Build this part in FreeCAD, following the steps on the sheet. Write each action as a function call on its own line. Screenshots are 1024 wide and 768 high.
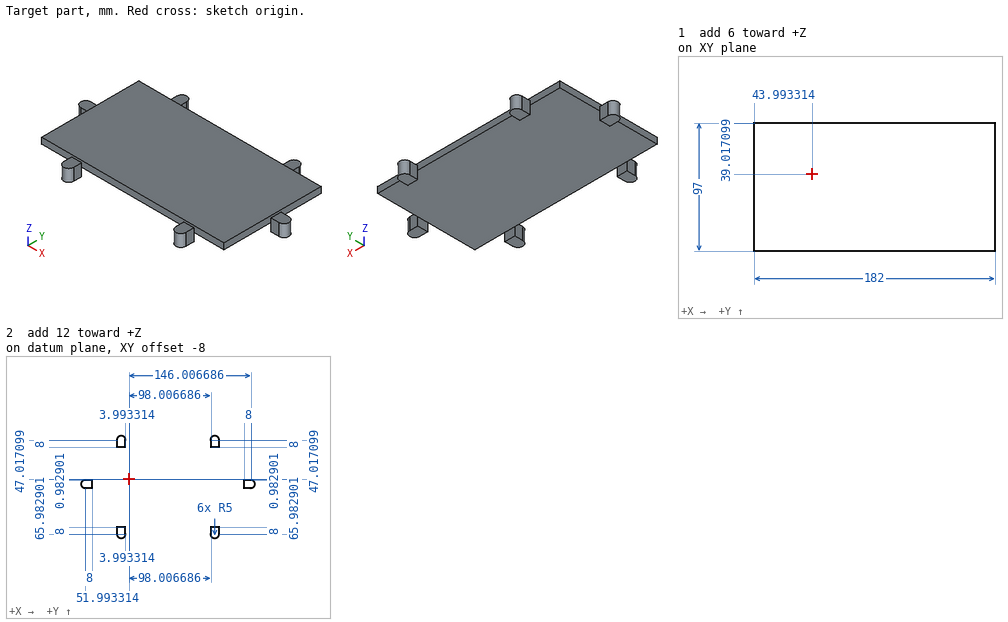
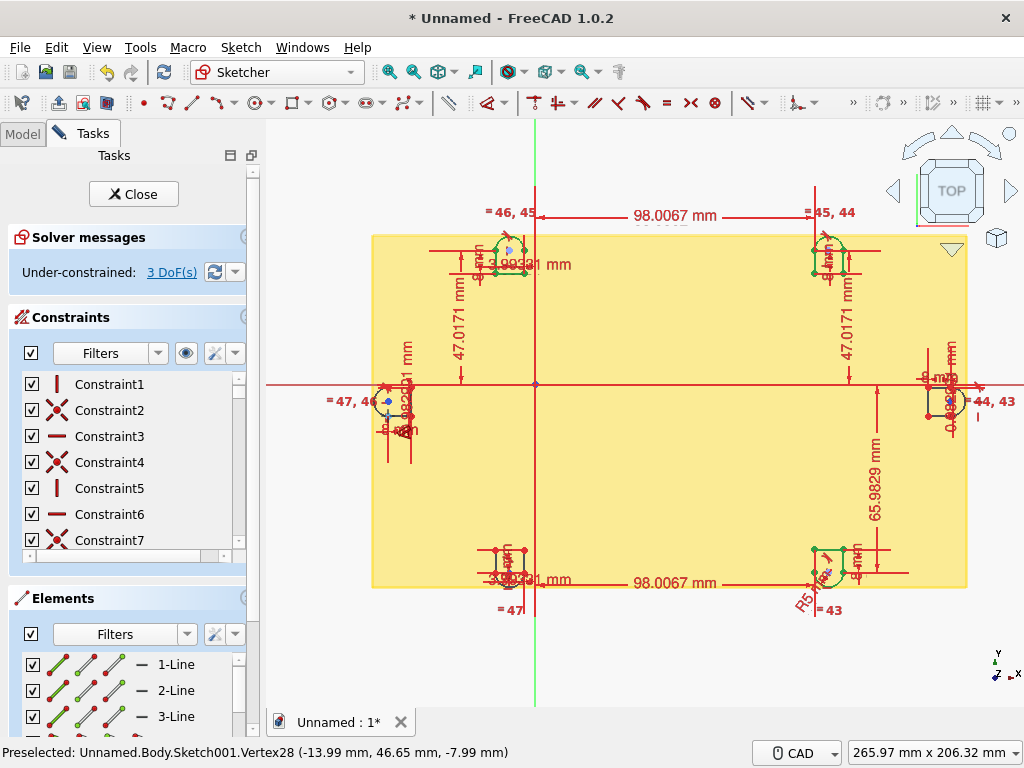
click(388, 416)
click(462, 351)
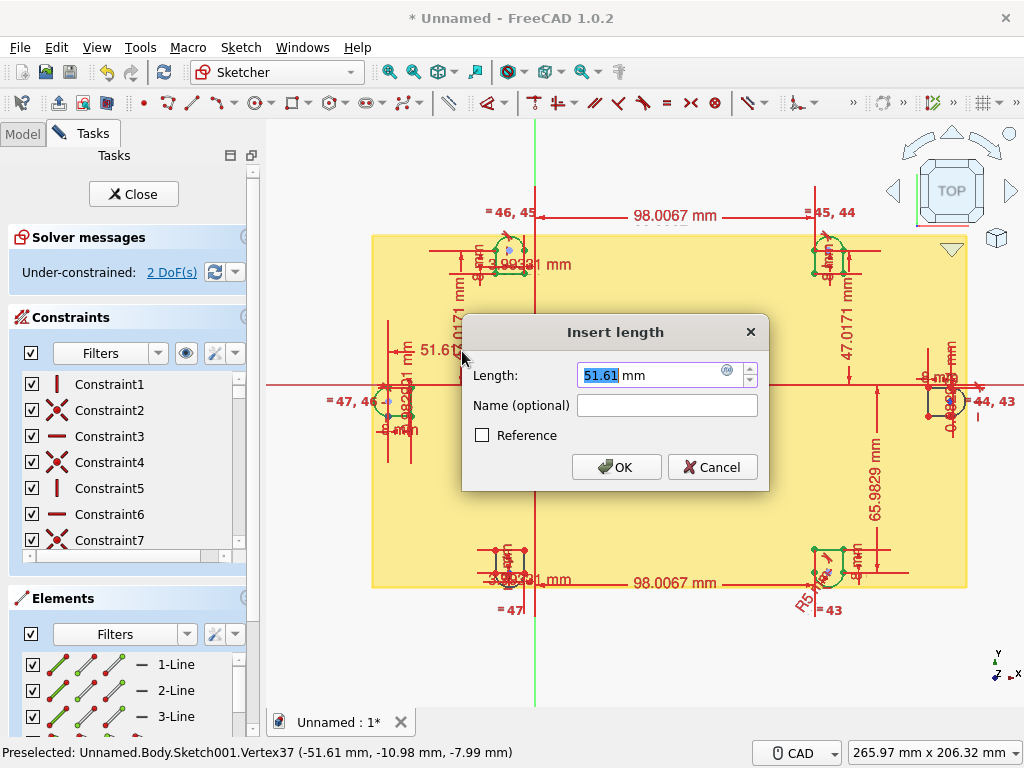
text(51.993314)
key(Return)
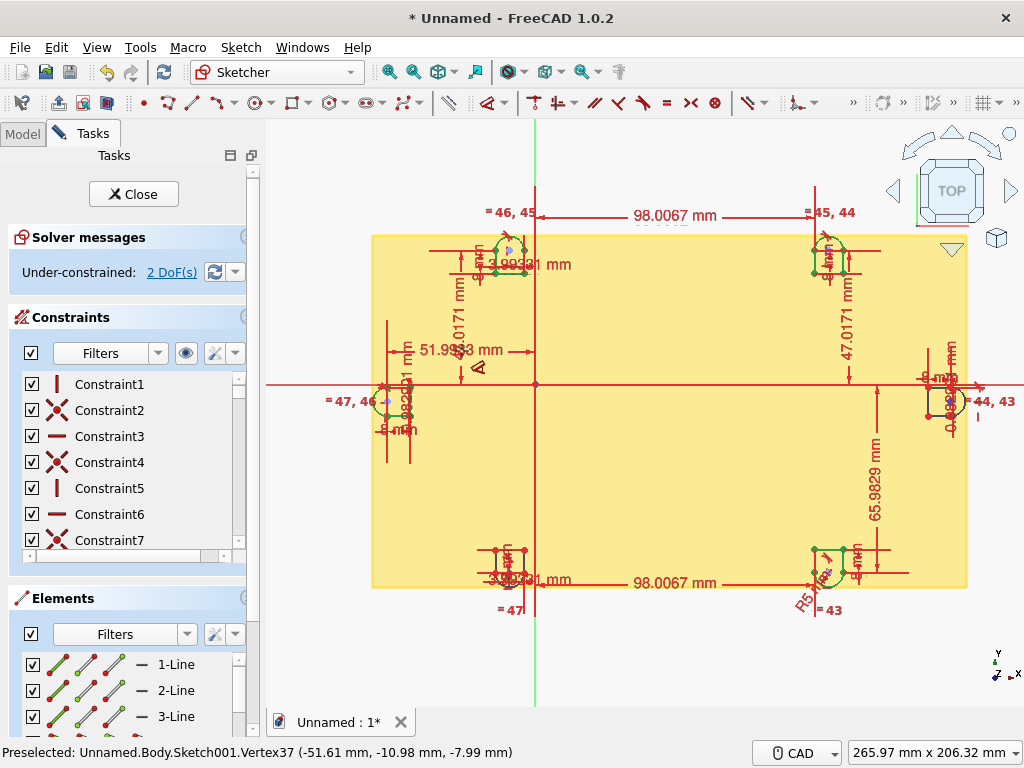
click(524, 573)
click(490, 479)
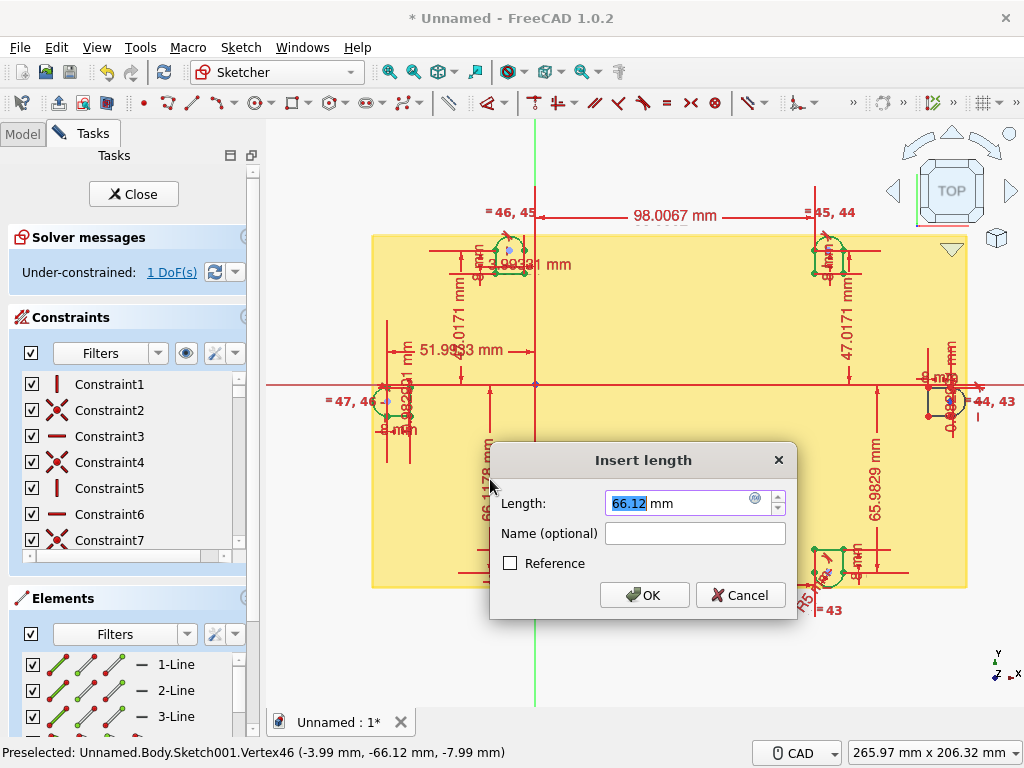
text(65.982901)
key(Return)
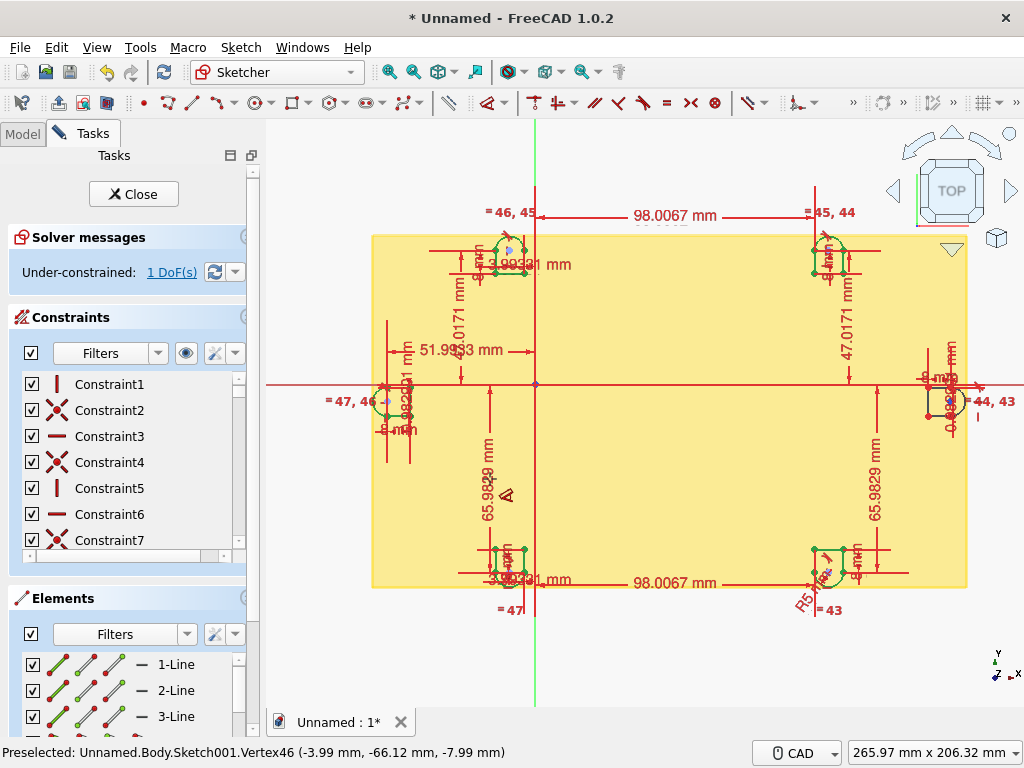
scroll(388, 416, down, 2)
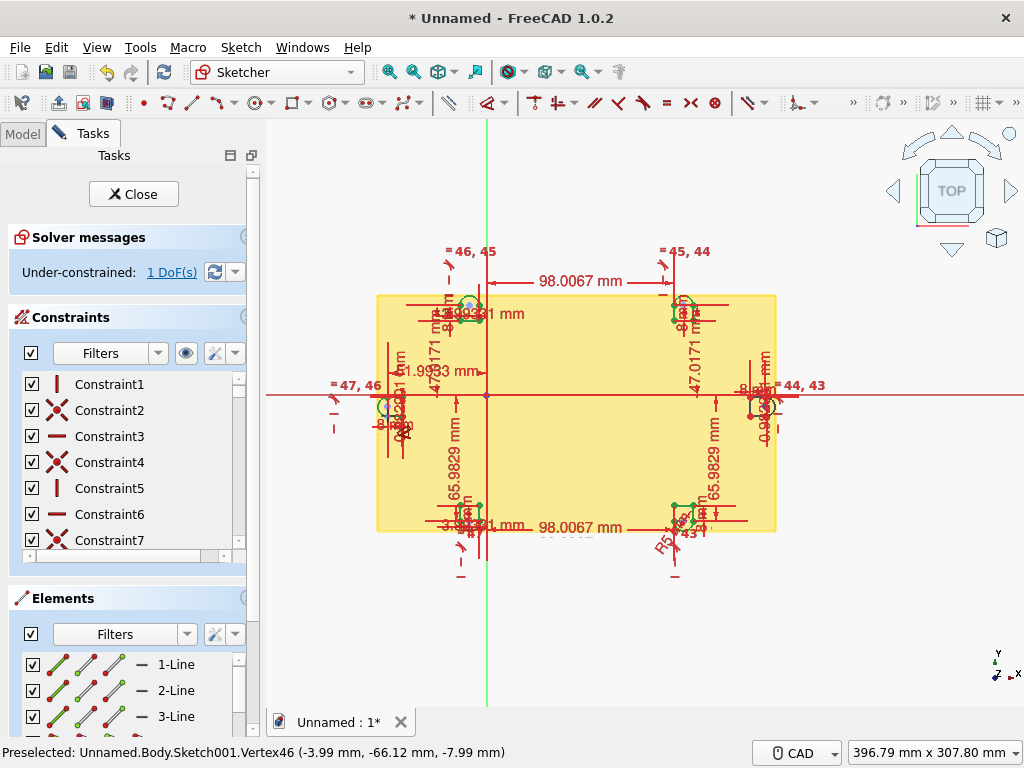
scroll(765, 397, up, 2)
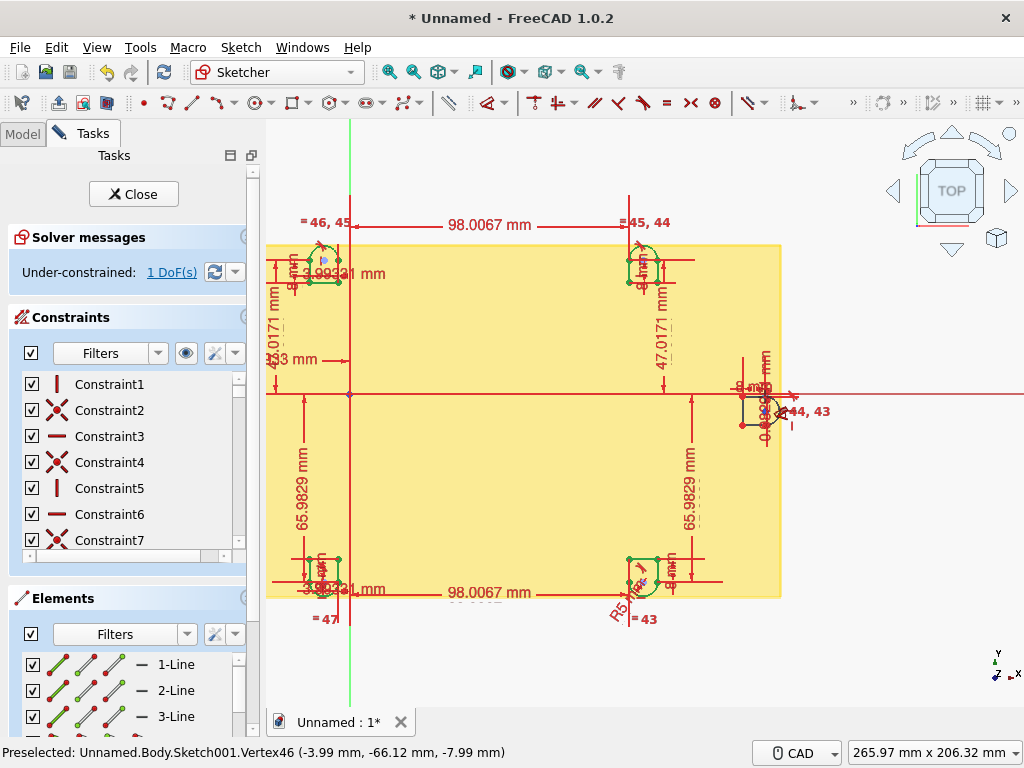
click(765, 397)
click(558, 360)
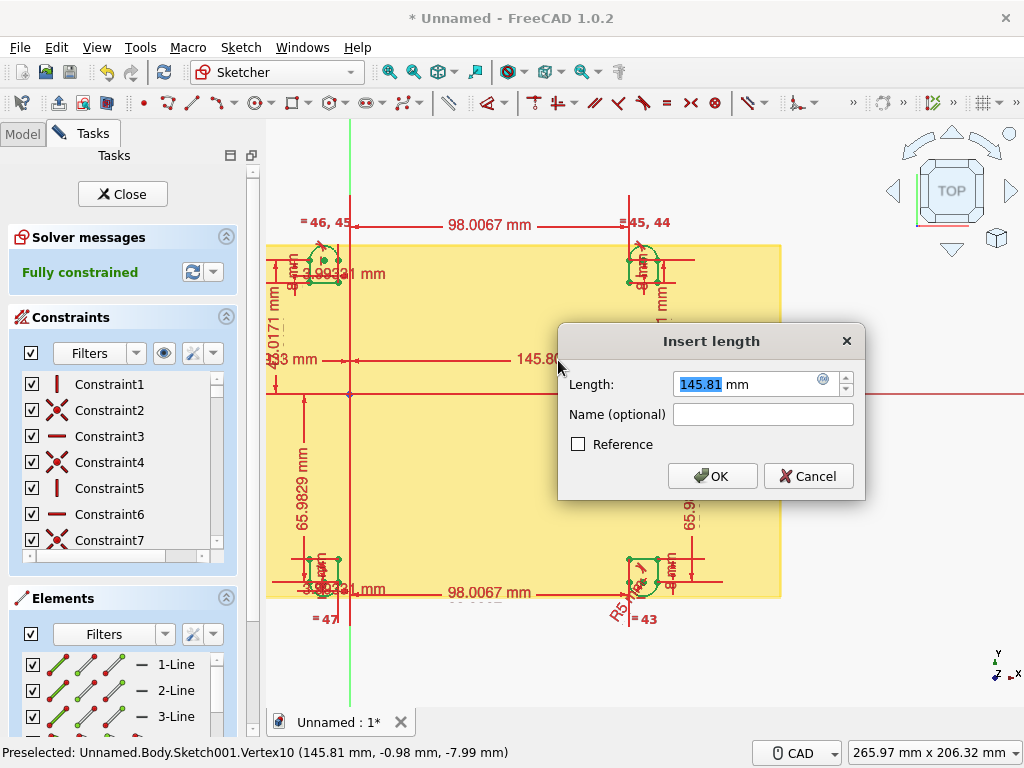
text(146.006686)
key(Return)
key(Escape)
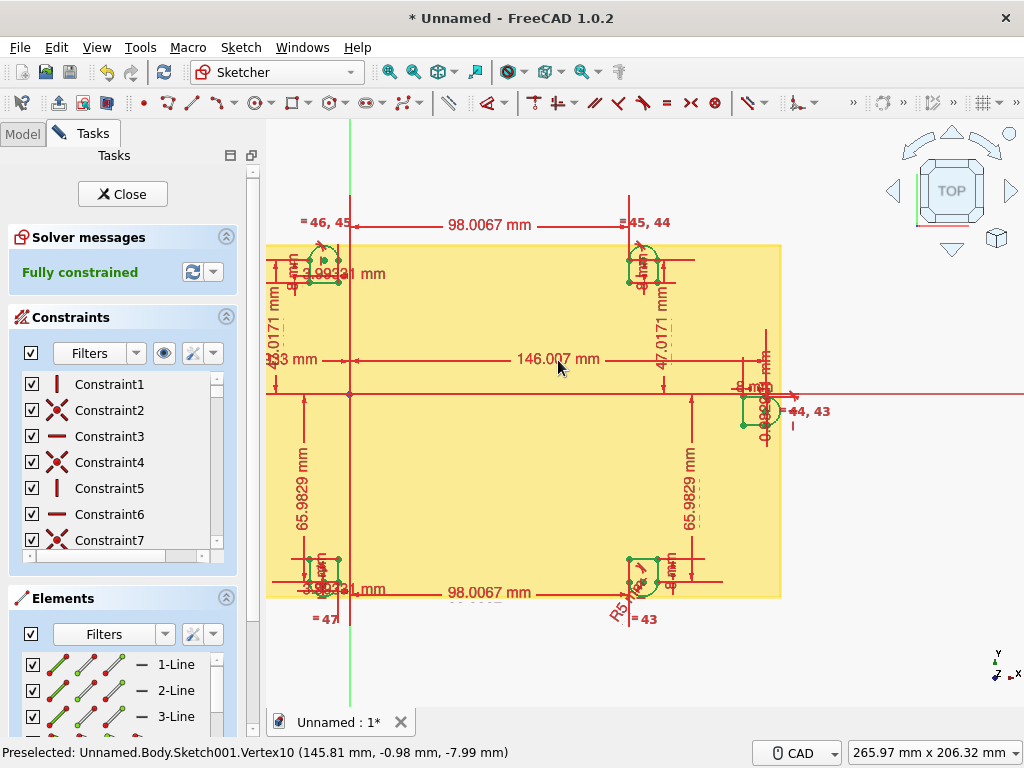
click(123, 194)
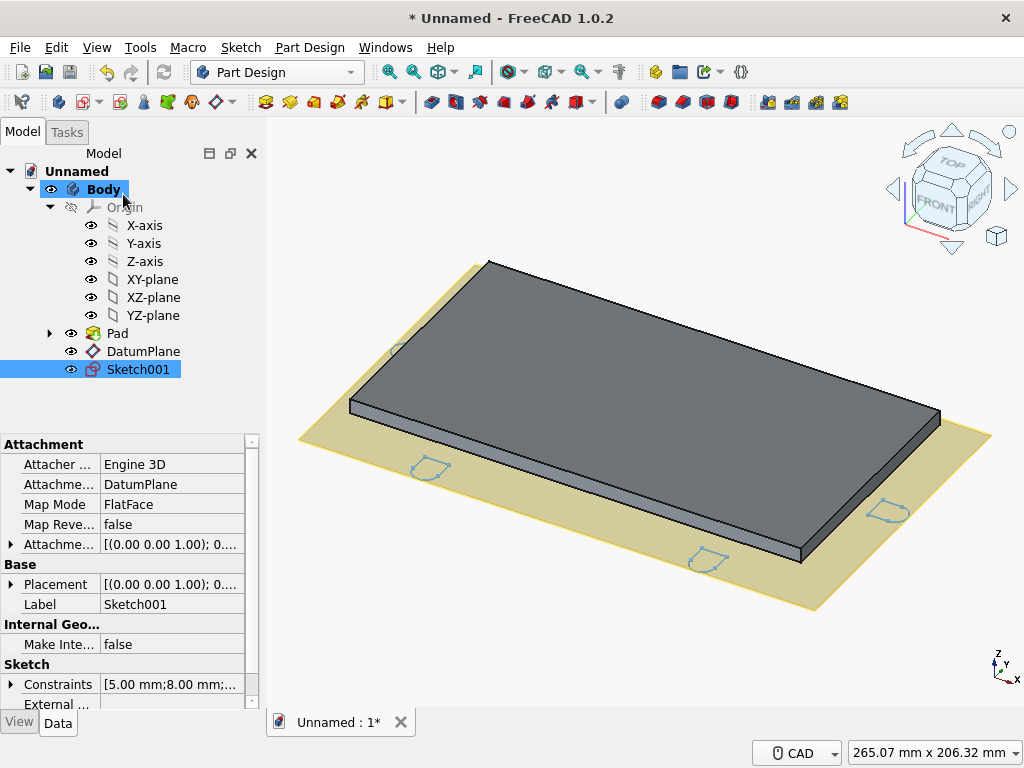
click(266, 102)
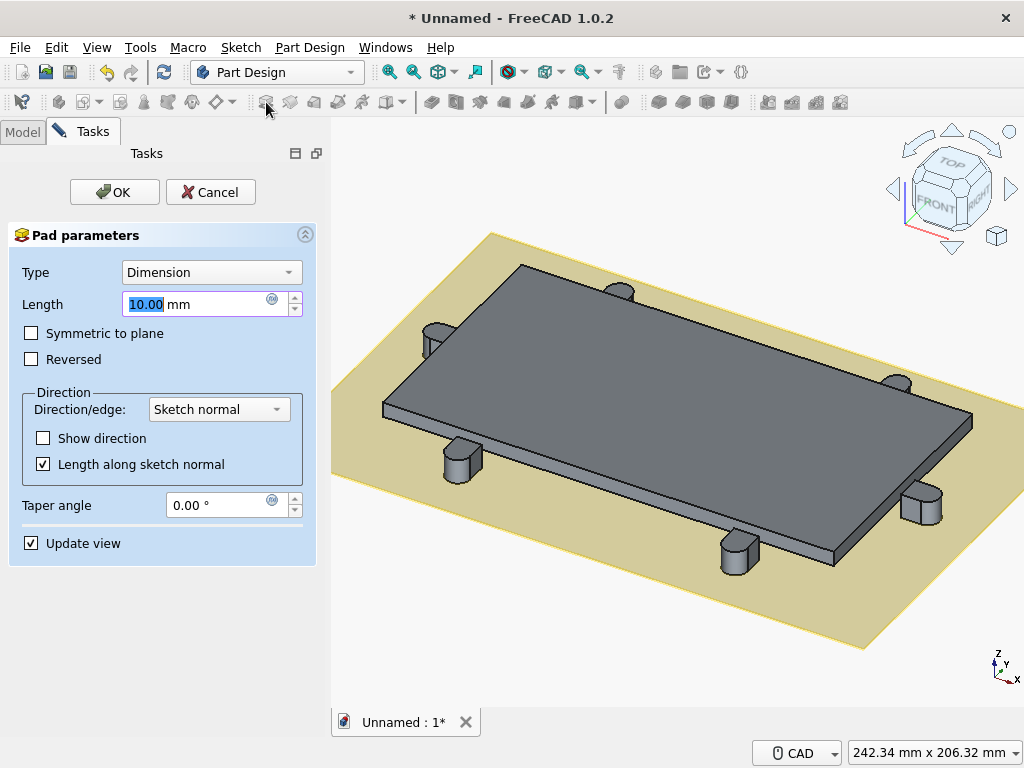
text(12)
key(Tab)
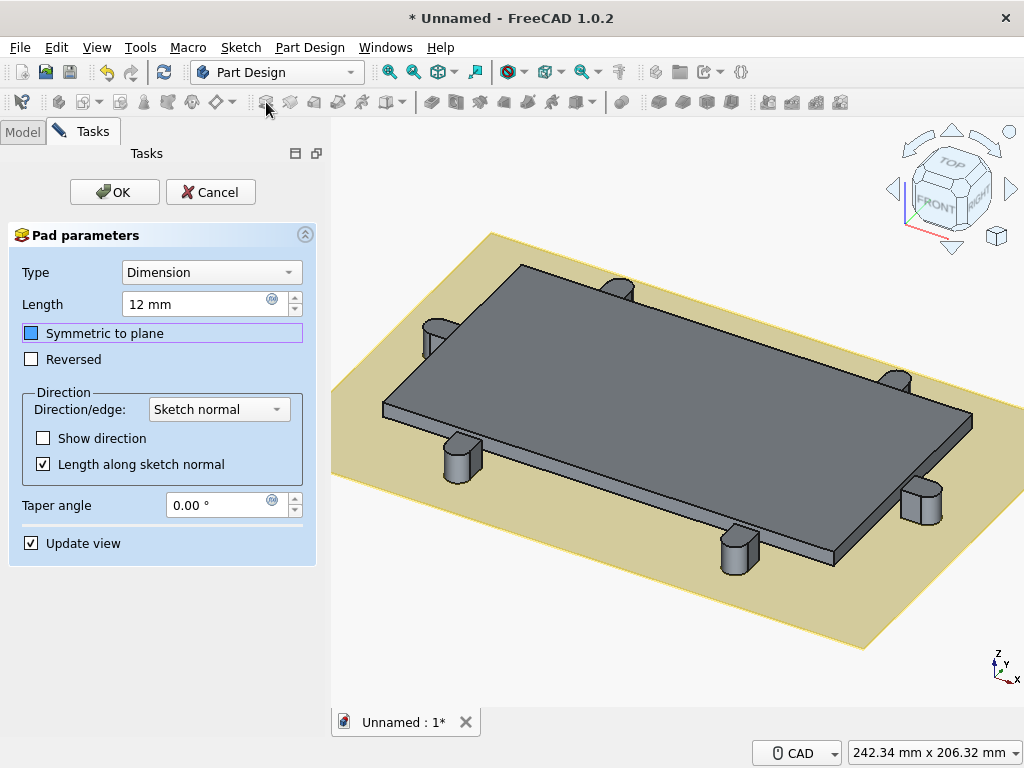
click(115, 192)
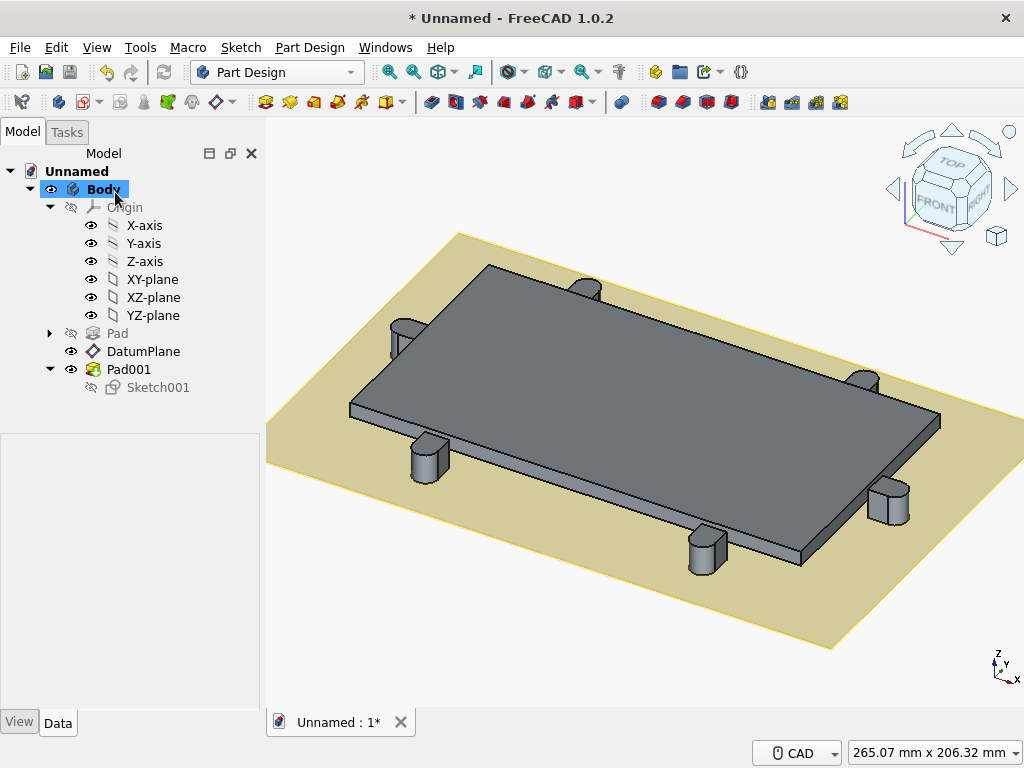
click(116, 351)
key(space)